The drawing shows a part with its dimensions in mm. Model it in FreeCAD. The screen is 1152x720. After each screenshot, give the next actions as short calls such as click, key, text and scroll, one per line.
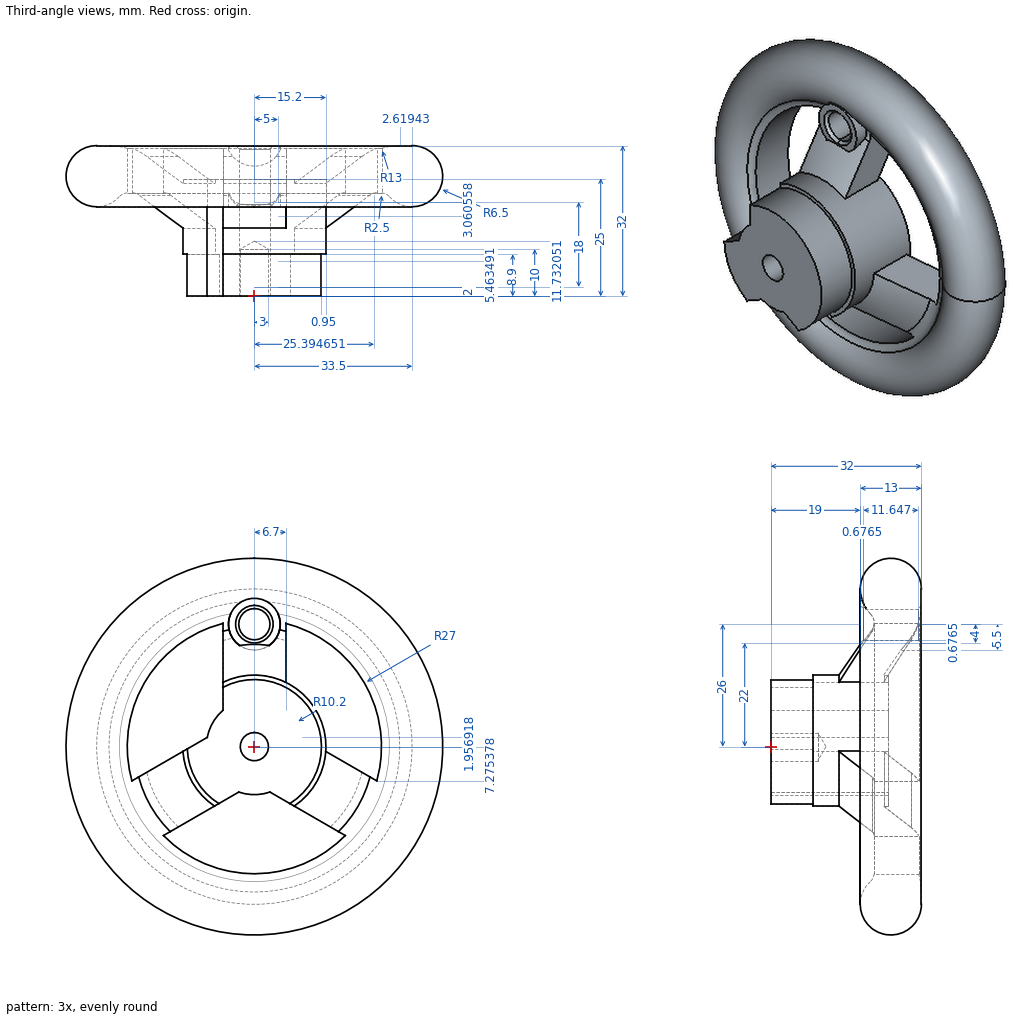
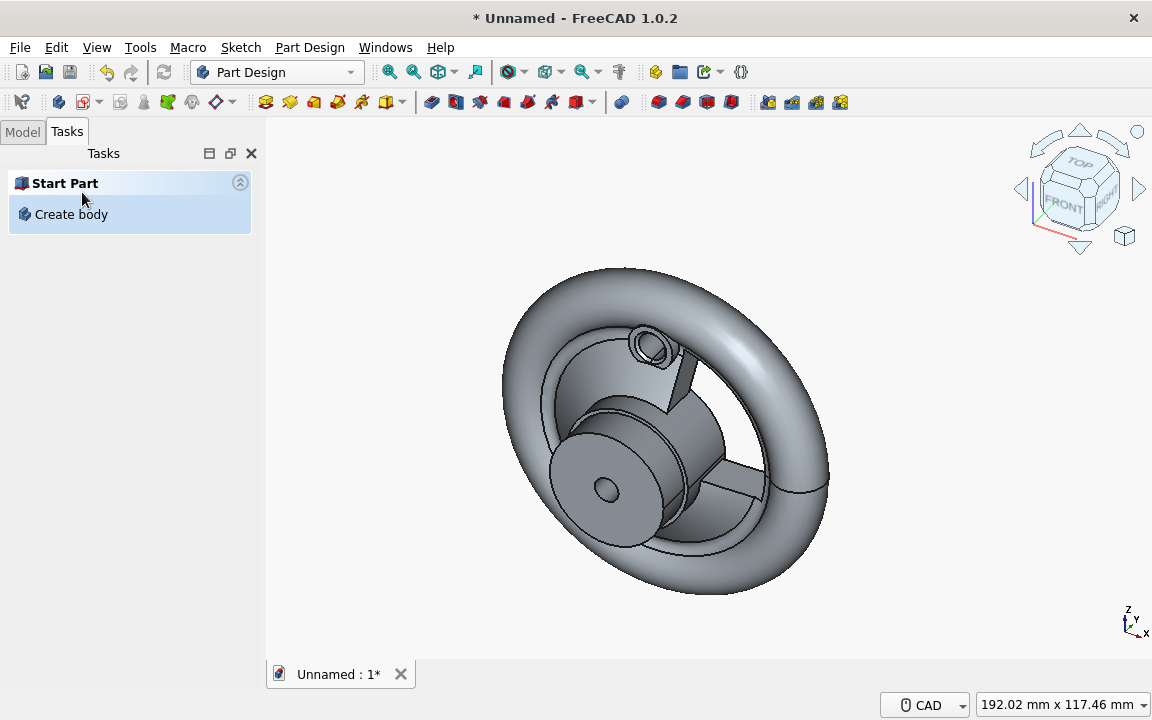
click(390, 72)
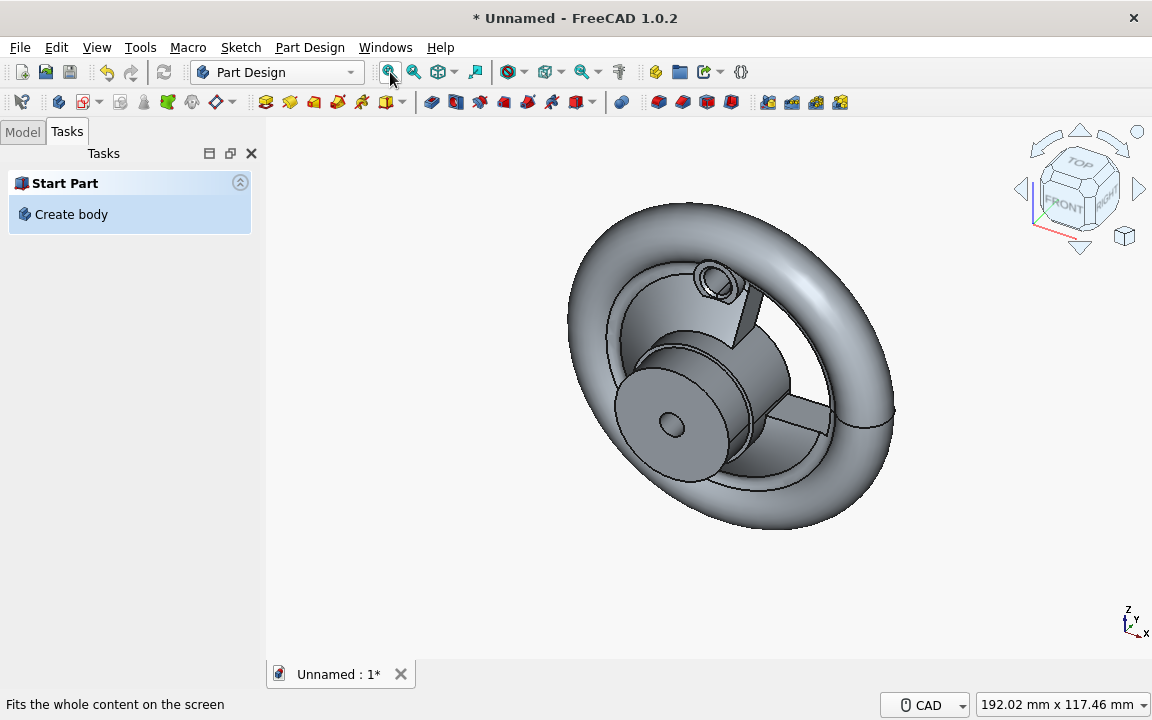
click(23, 131)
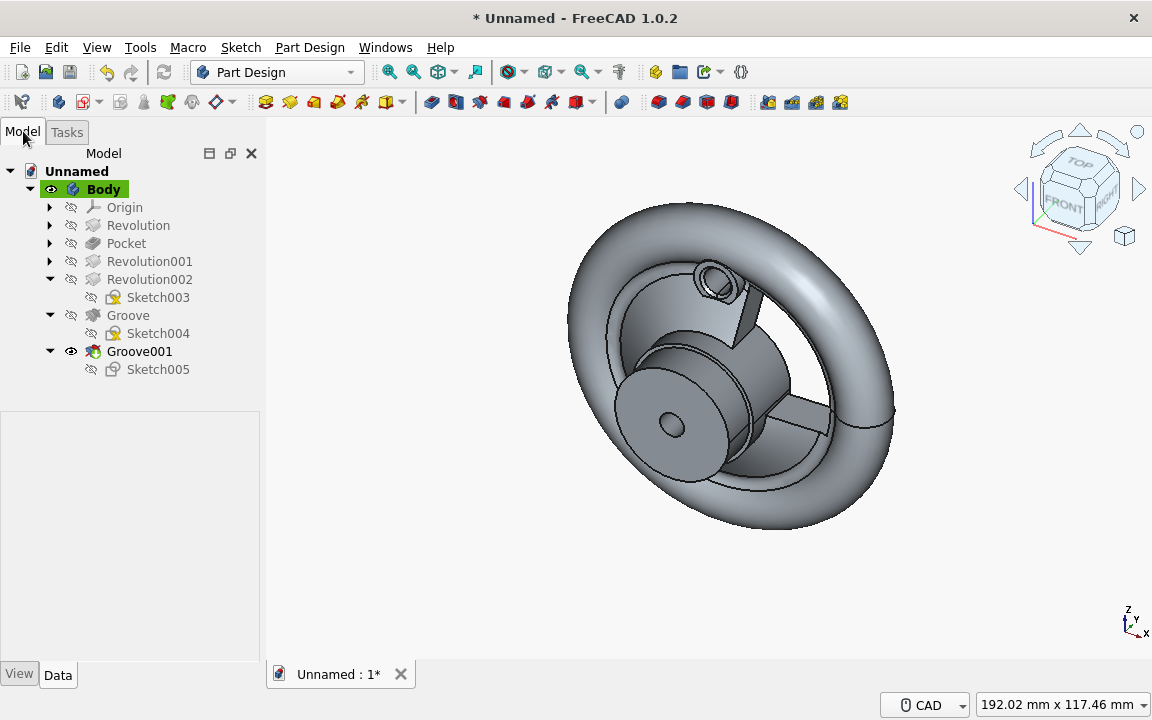
click(116, 243)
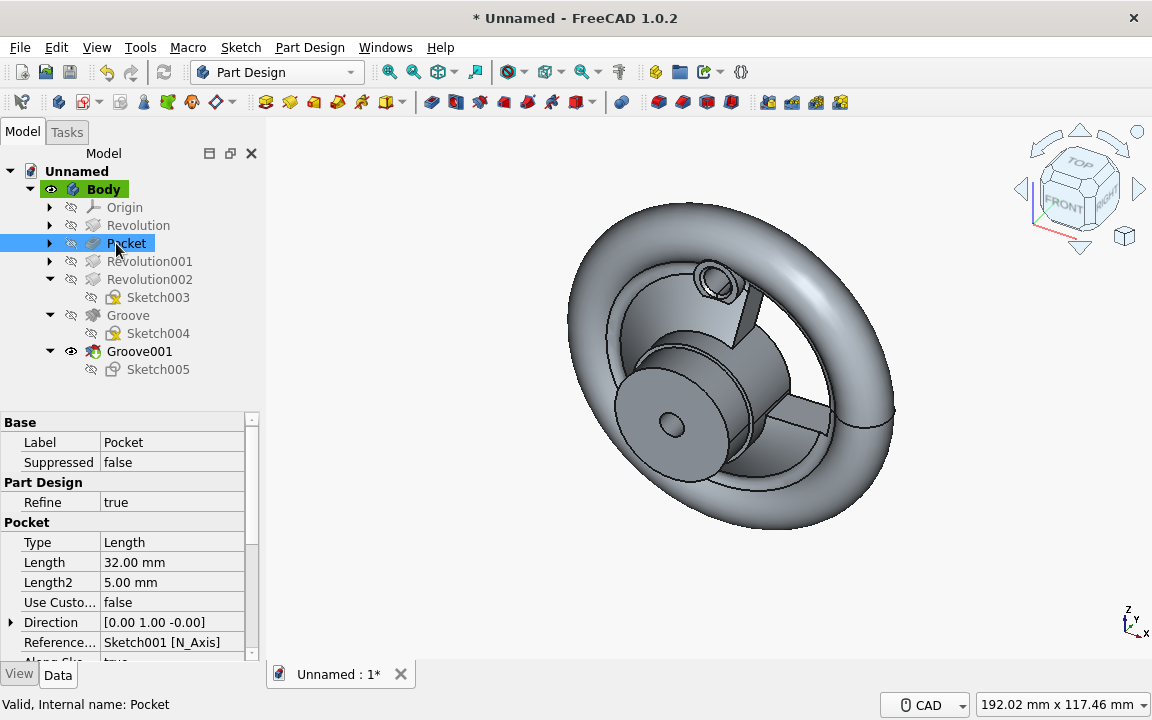
click(816, 102)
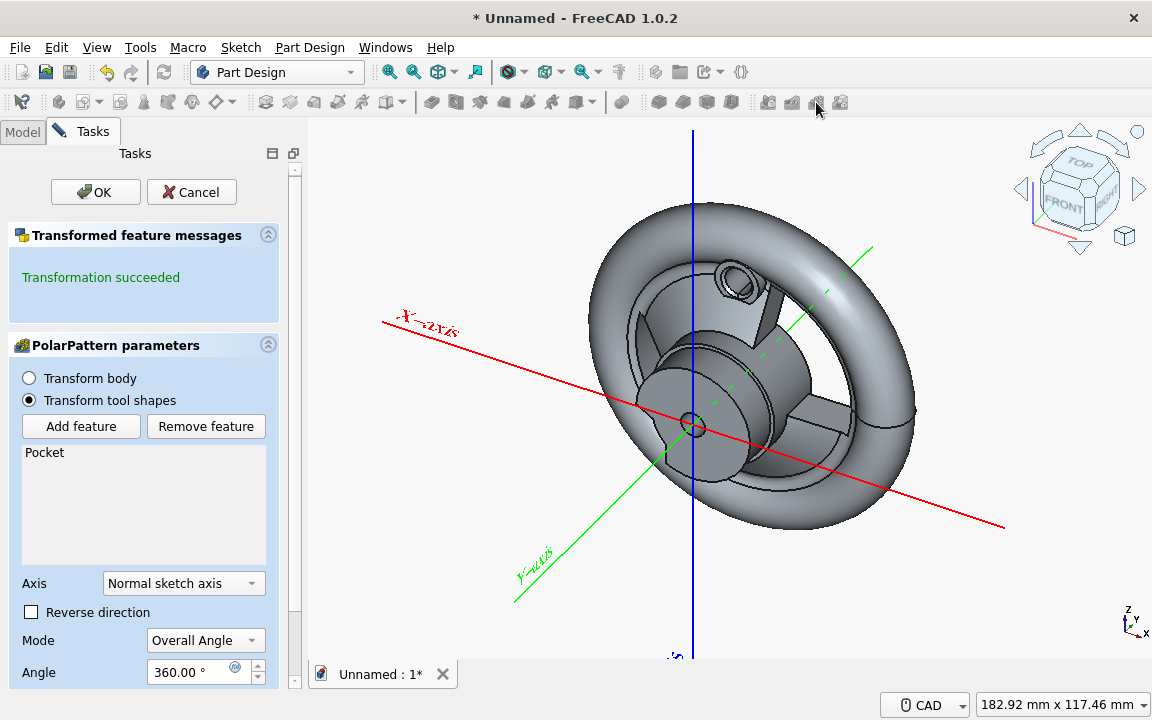
click(184, 584)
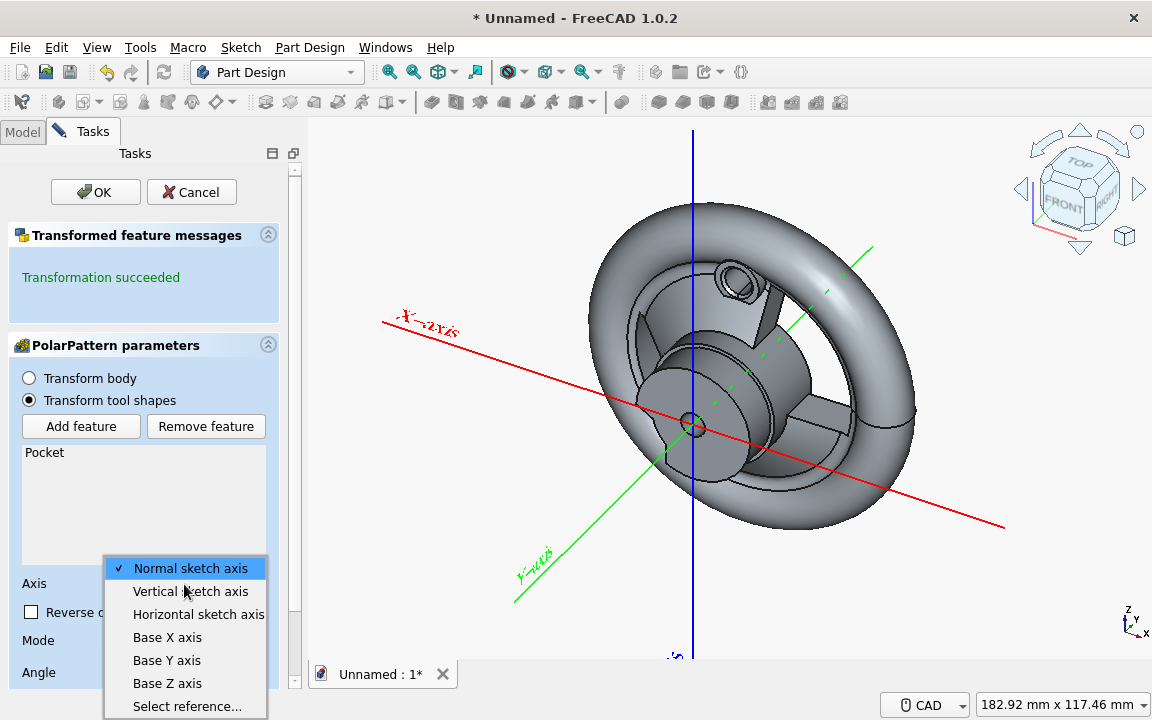
click(184, 660)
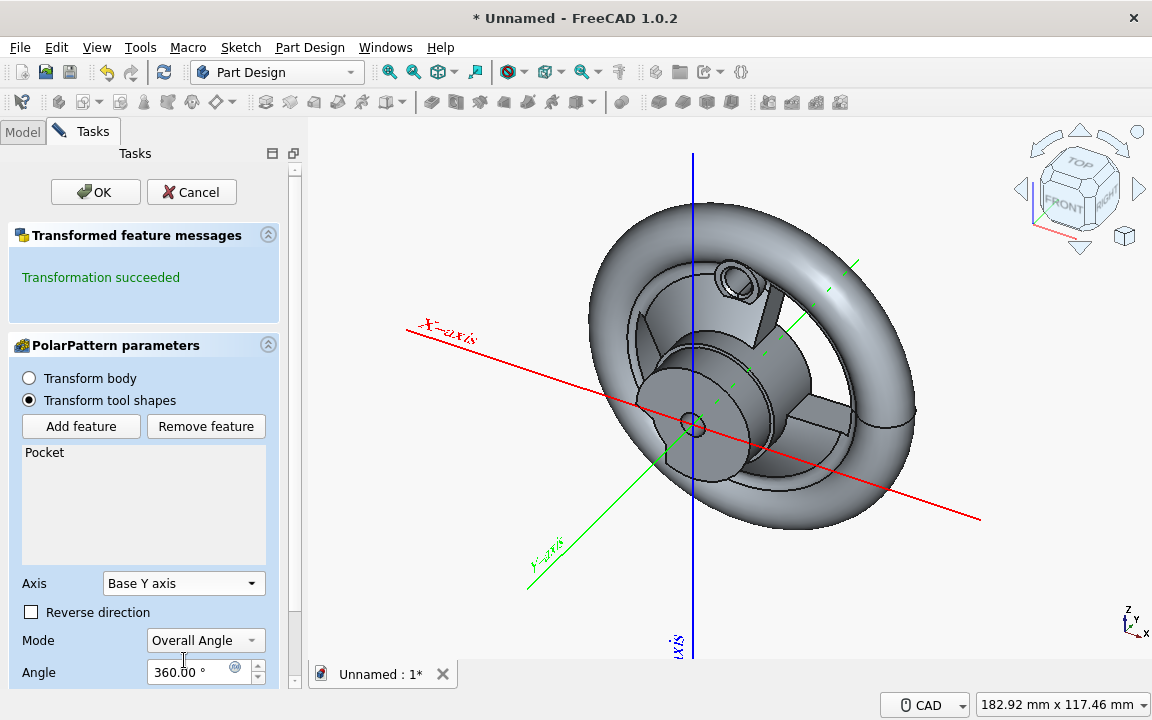
scroll(295, 426, down, 2)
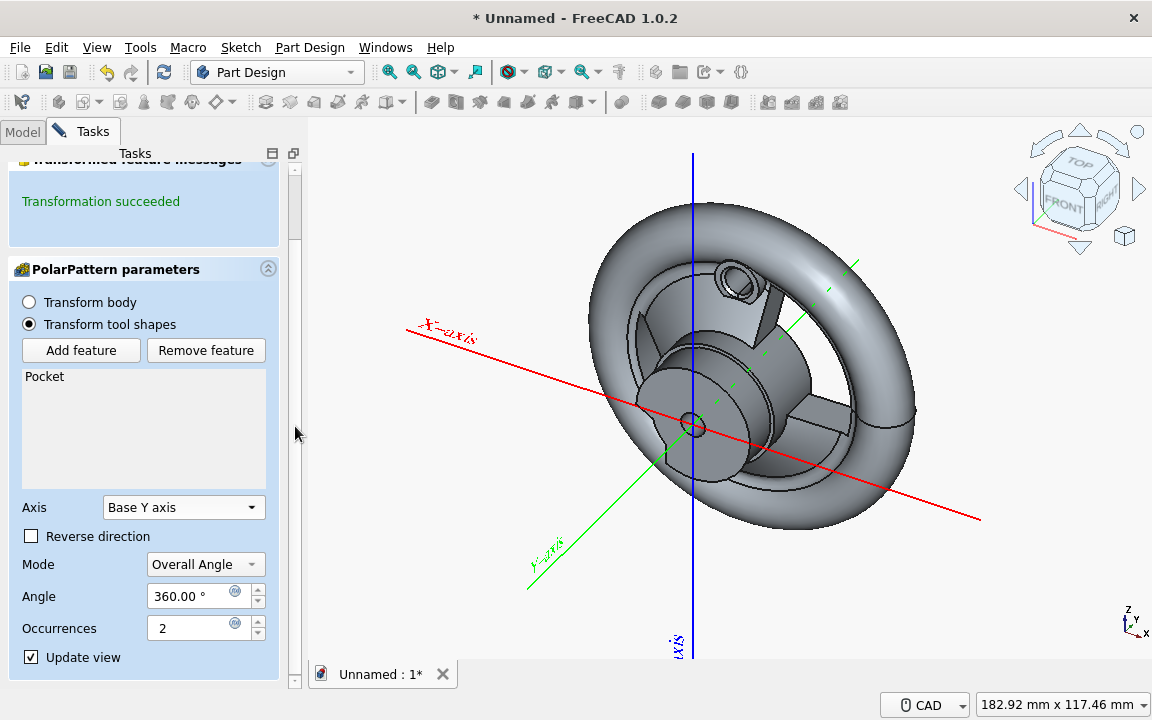
triple_click(198, 628)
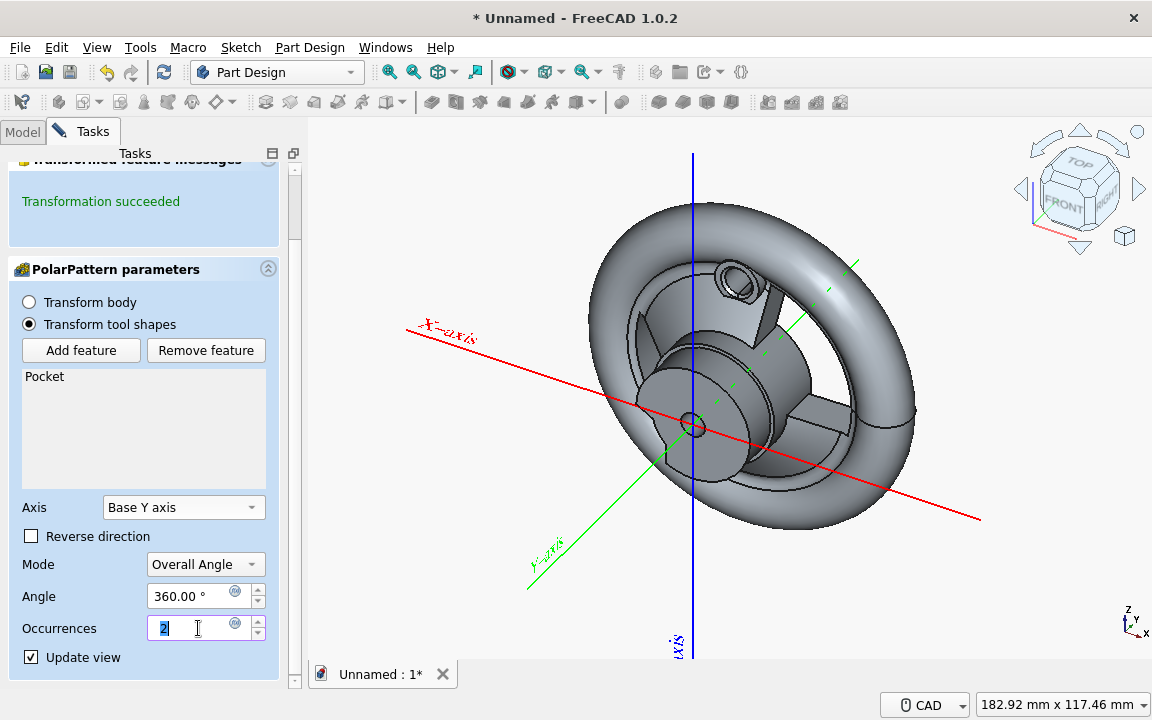
text(3)
key(Tab)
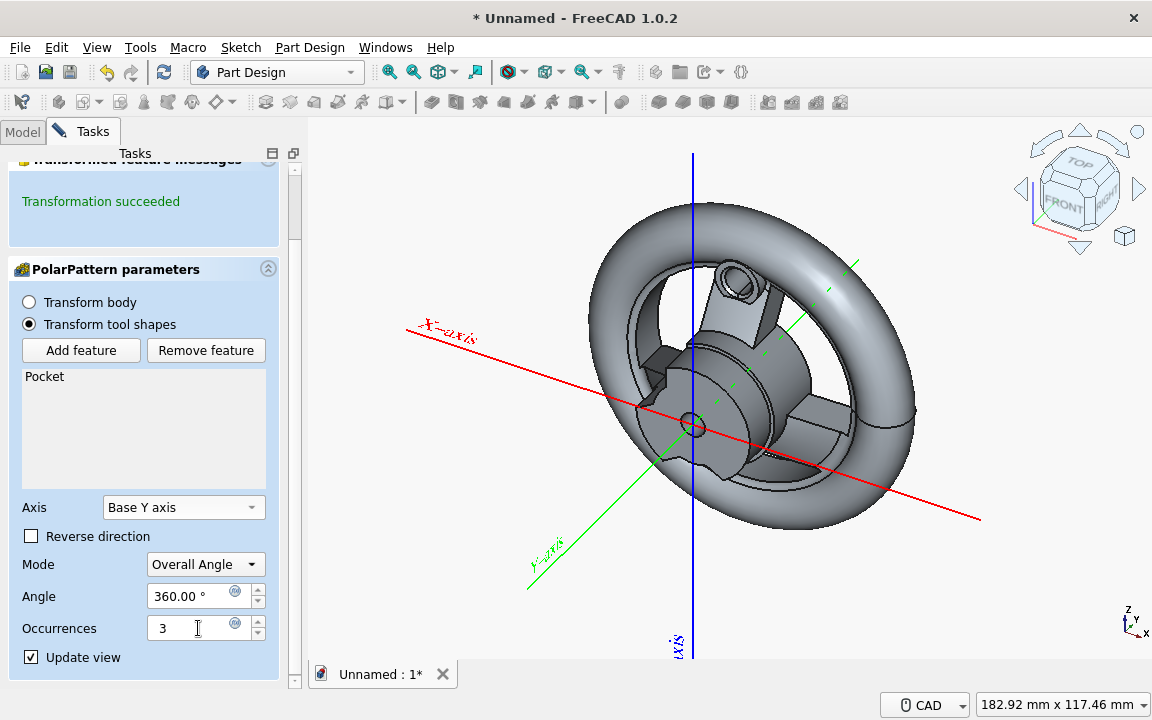
scroll(295, 426, up, 3)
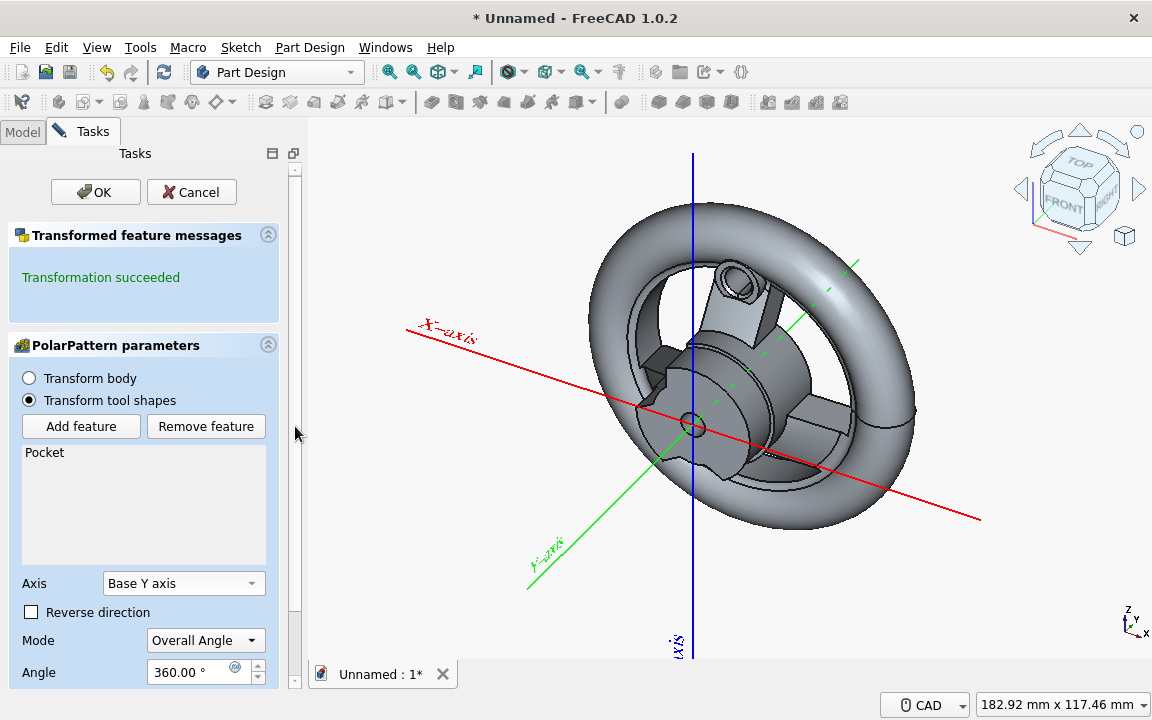
click(96, 192)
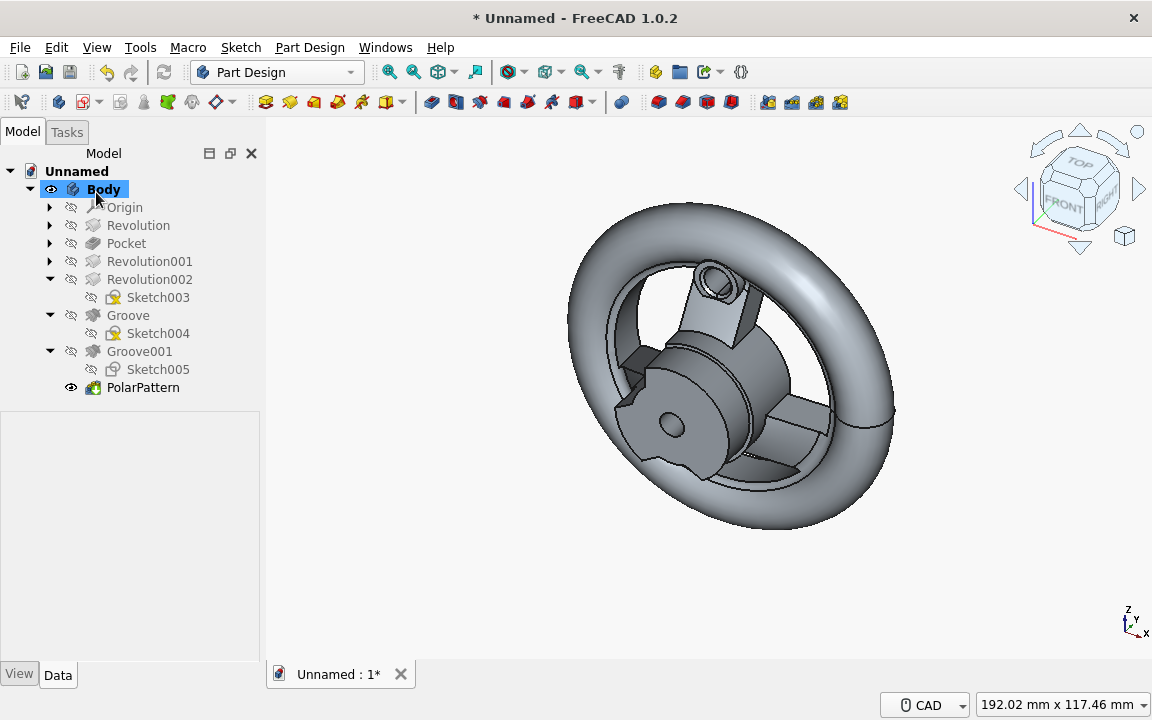
key(0)